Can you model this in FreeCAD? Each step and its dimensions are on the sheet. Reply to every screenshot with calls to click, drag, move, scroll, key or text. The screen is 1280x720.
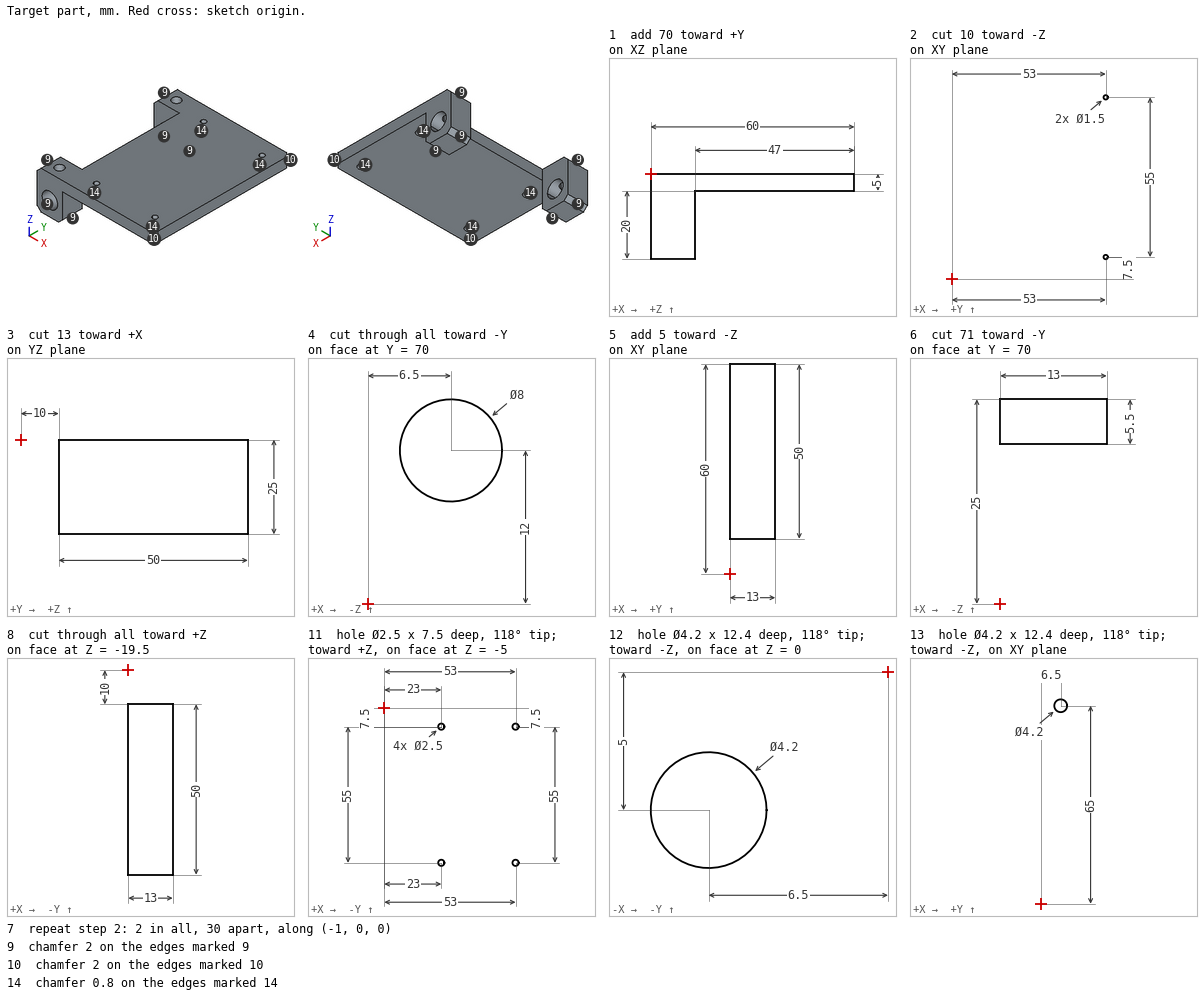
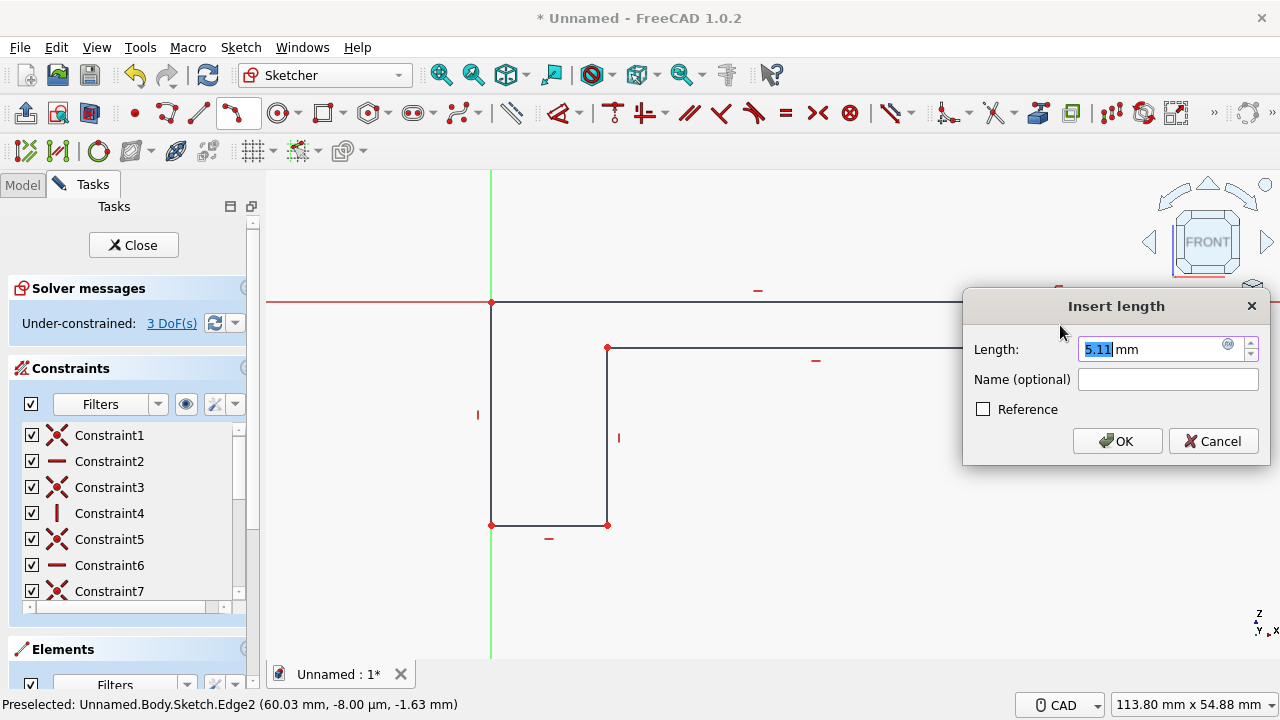
text(5)
key(Return)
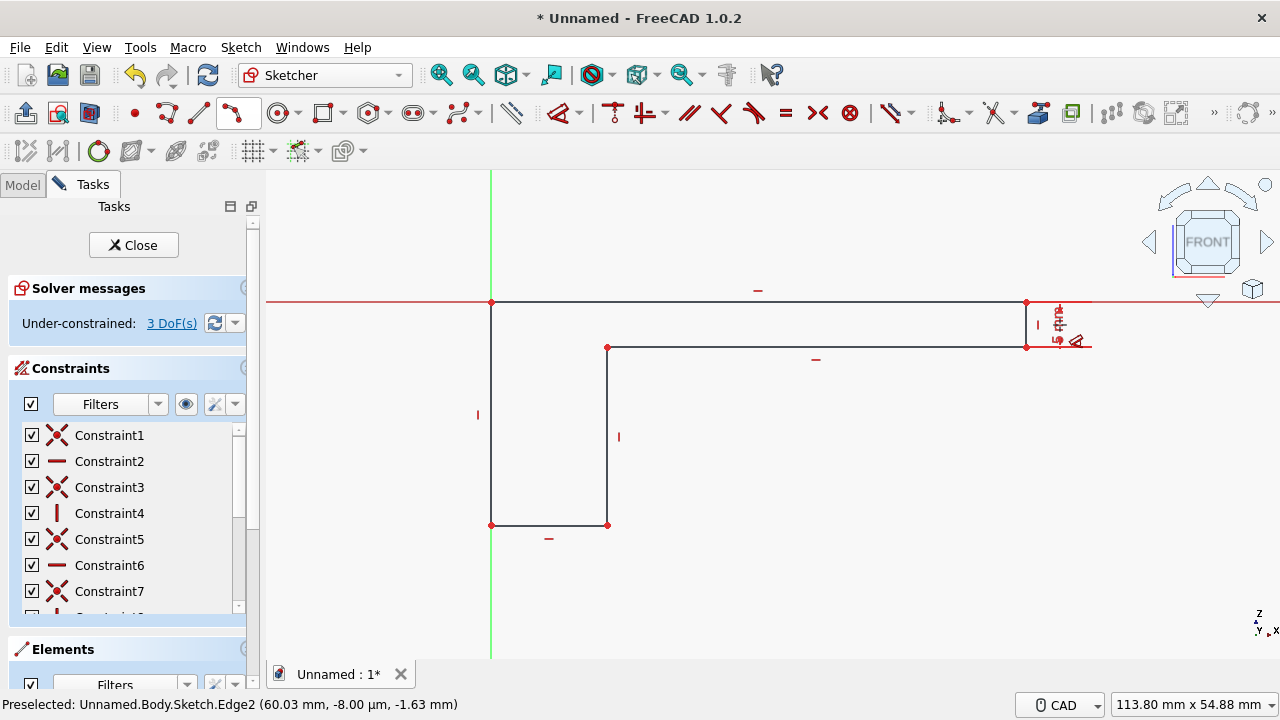
click(652, 302)
click(759, 268)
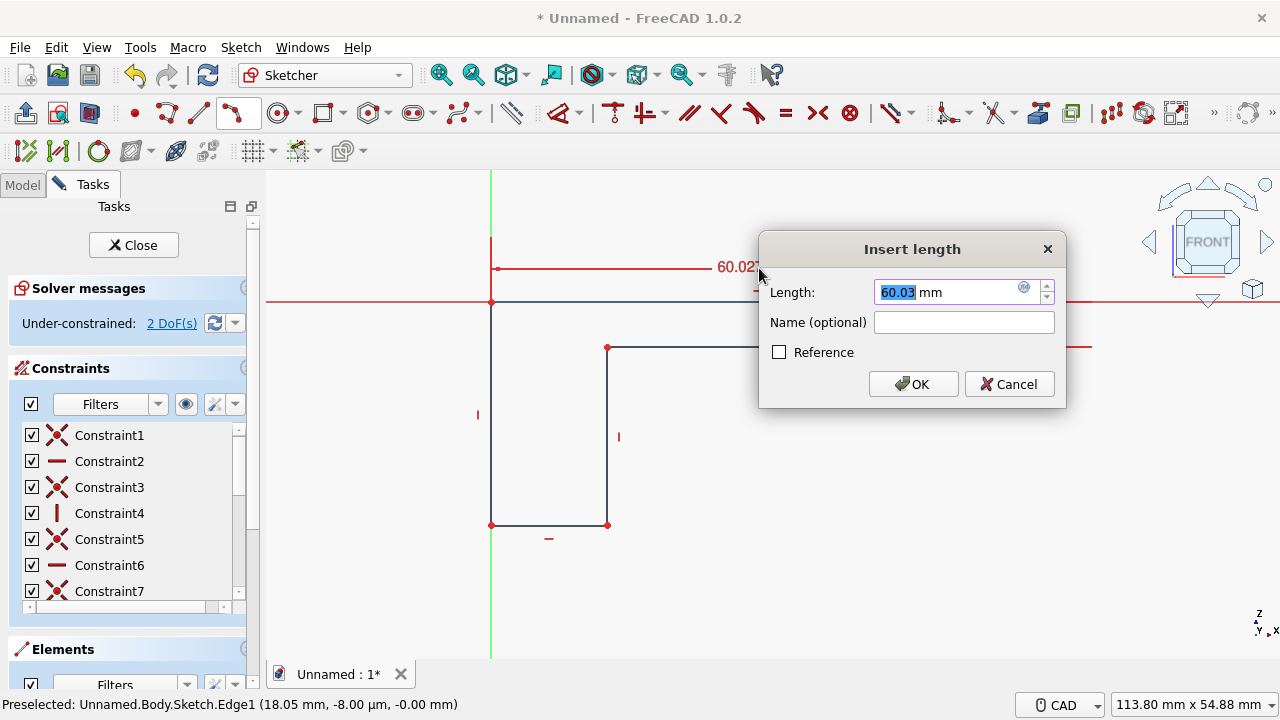
text(60)
key(Return)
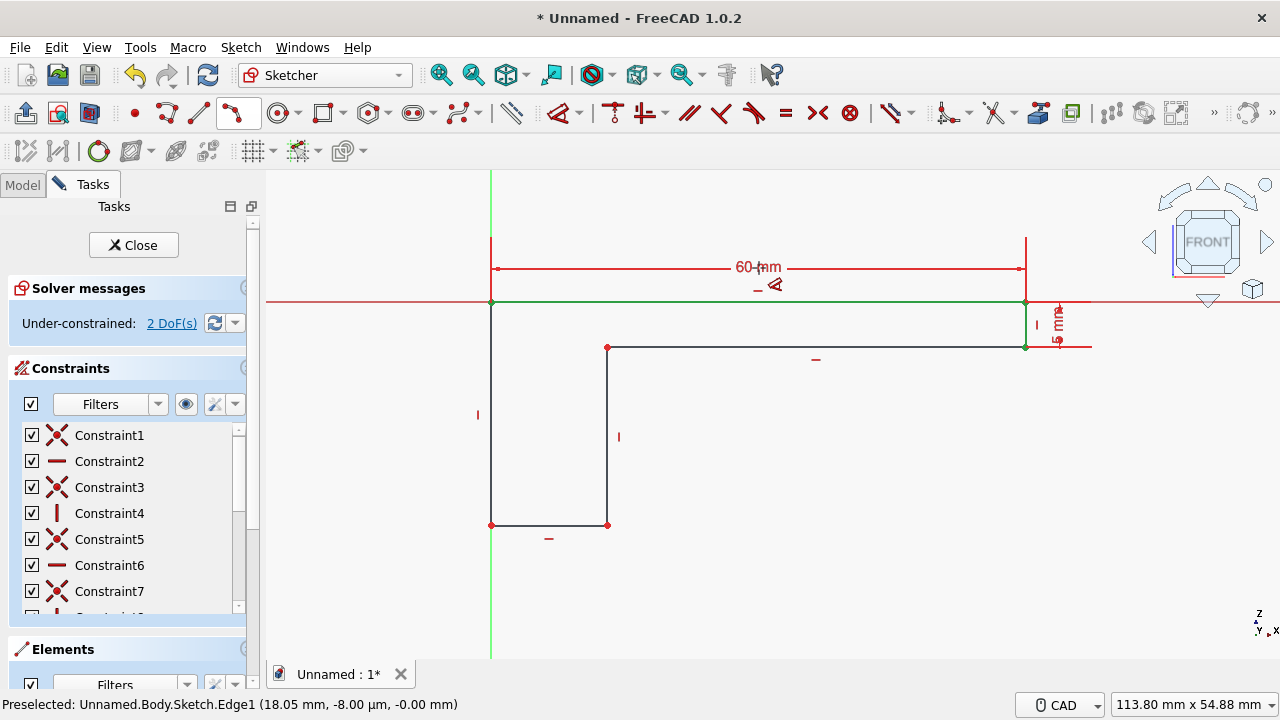
click(900, 347)
click(816, 381)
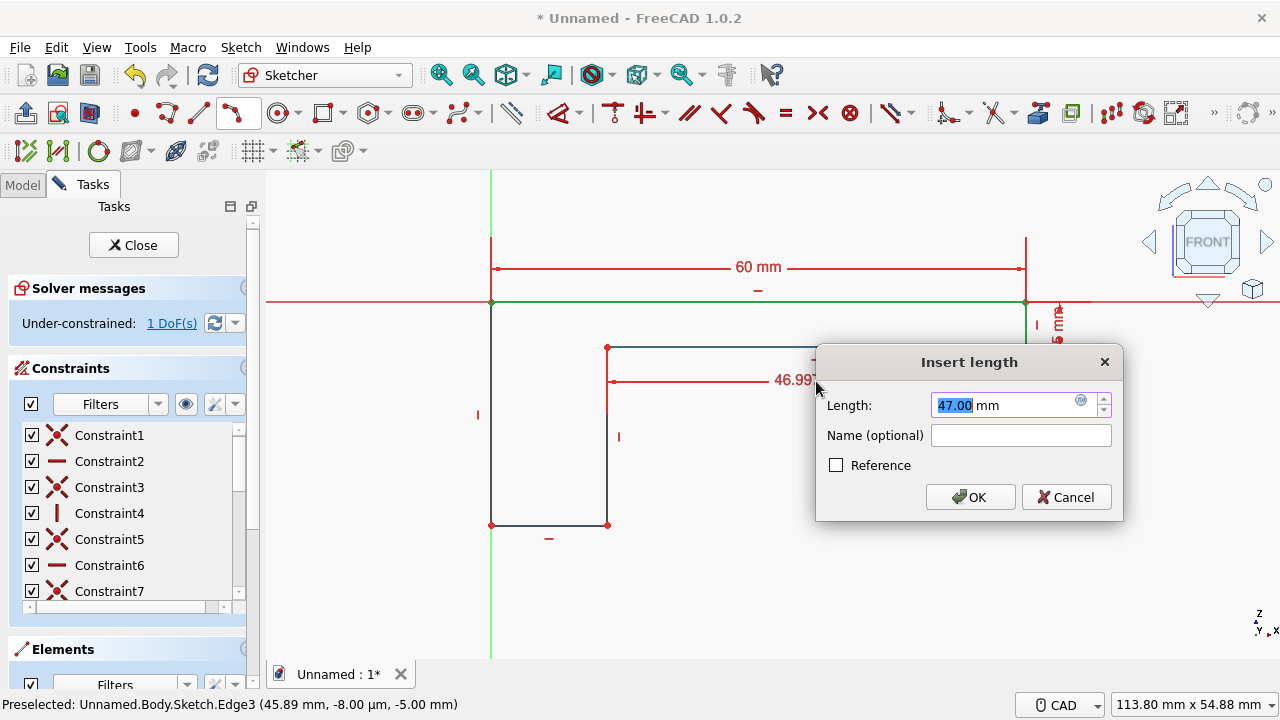
text(47)
key(Return)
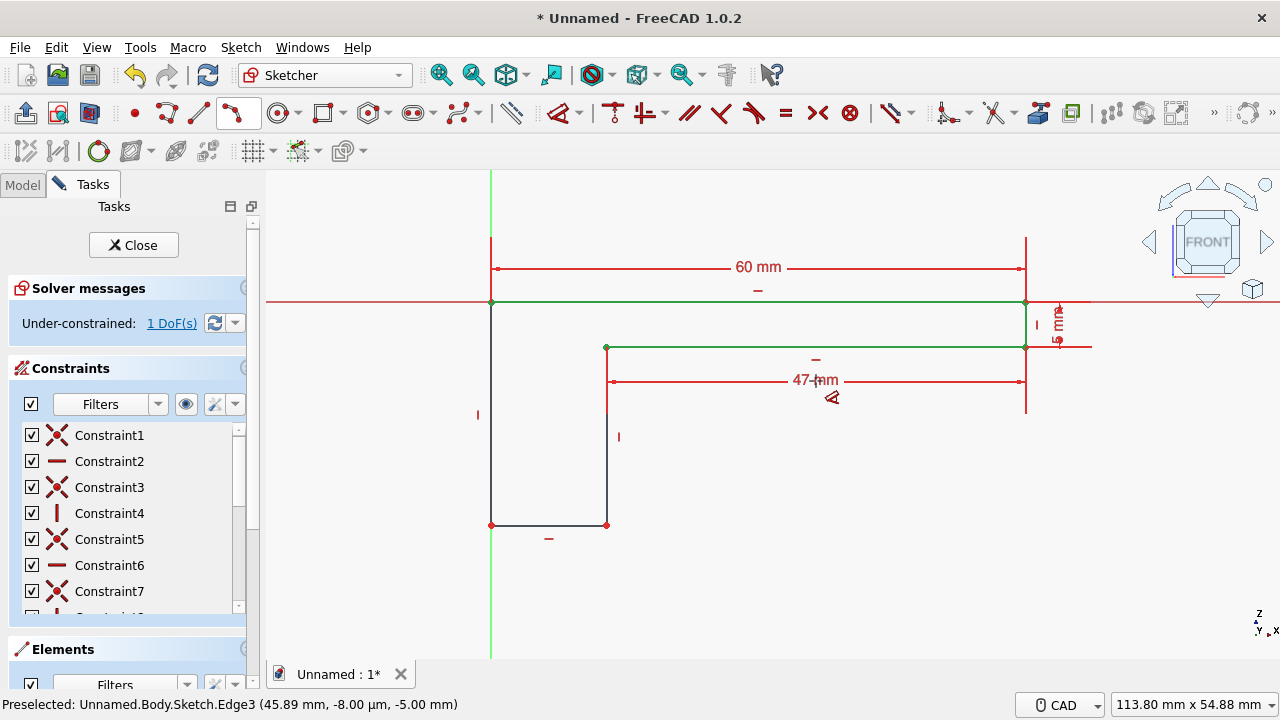
click(607, 401)
click(573, 437)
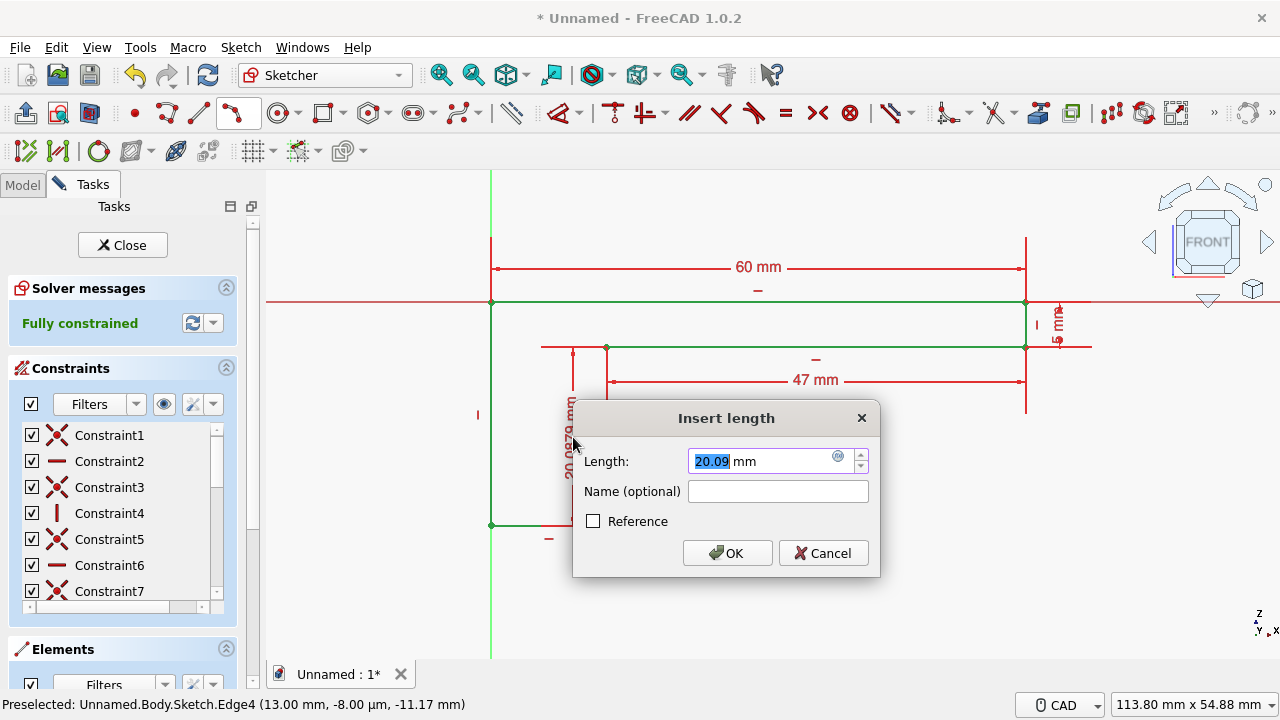
text(20)
key(Return)
key(Escape)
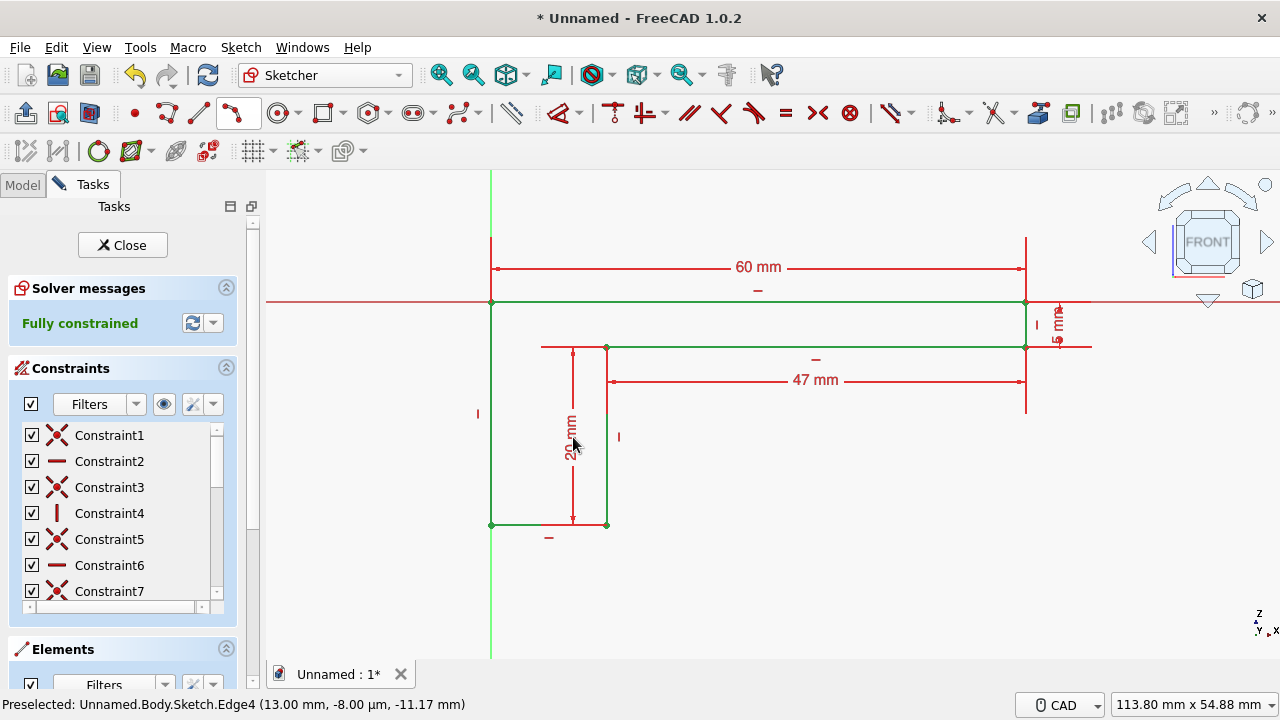
click(123, 245)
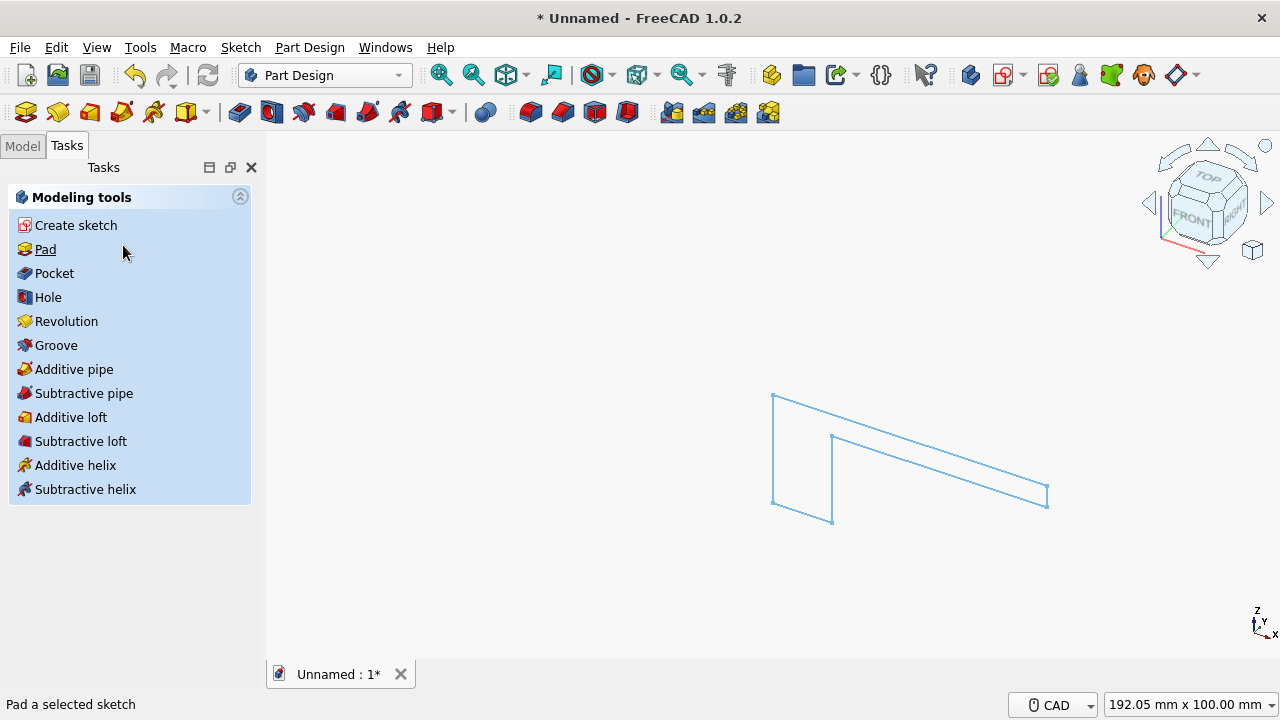
click(26, 112)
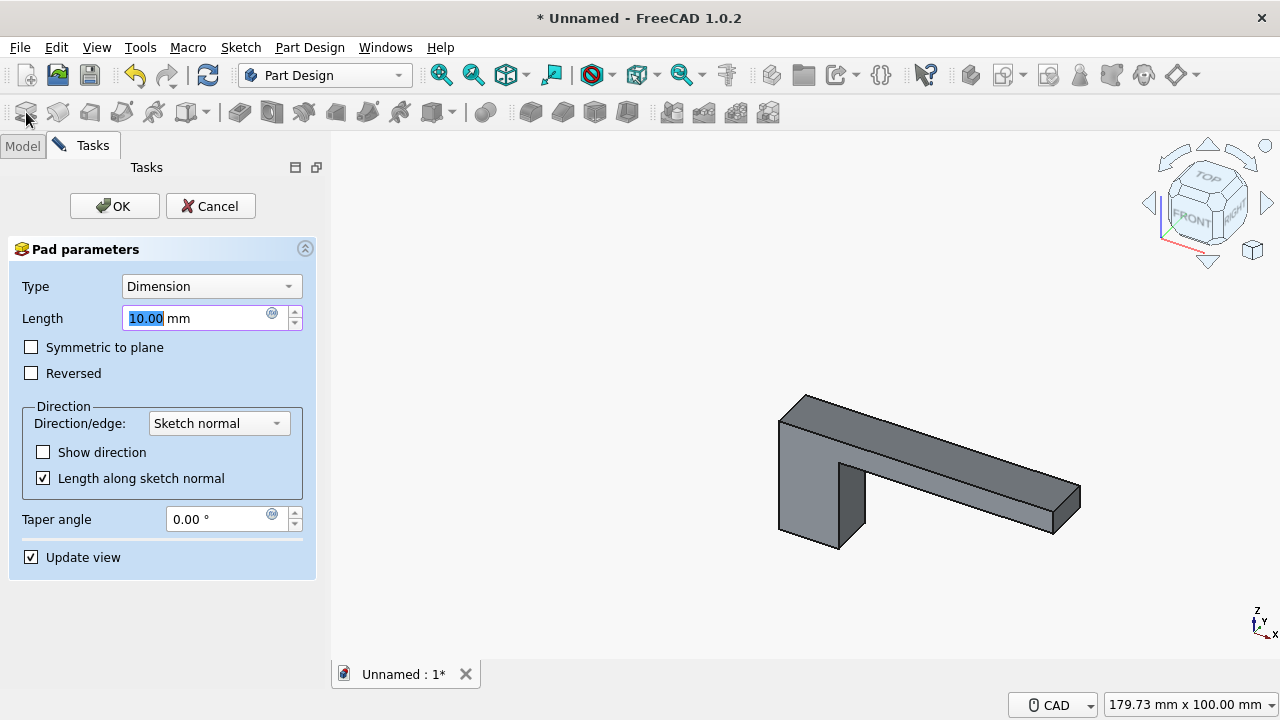
text(70)
key(Tab)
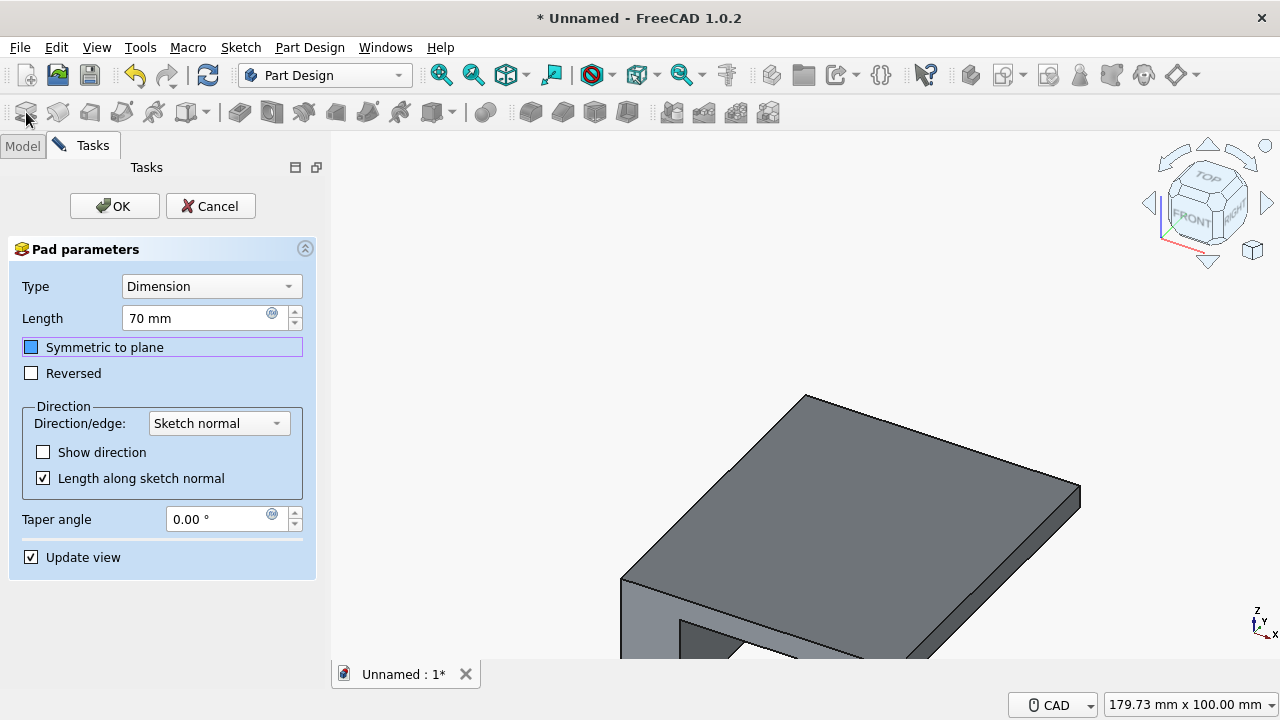
click(30, 373)